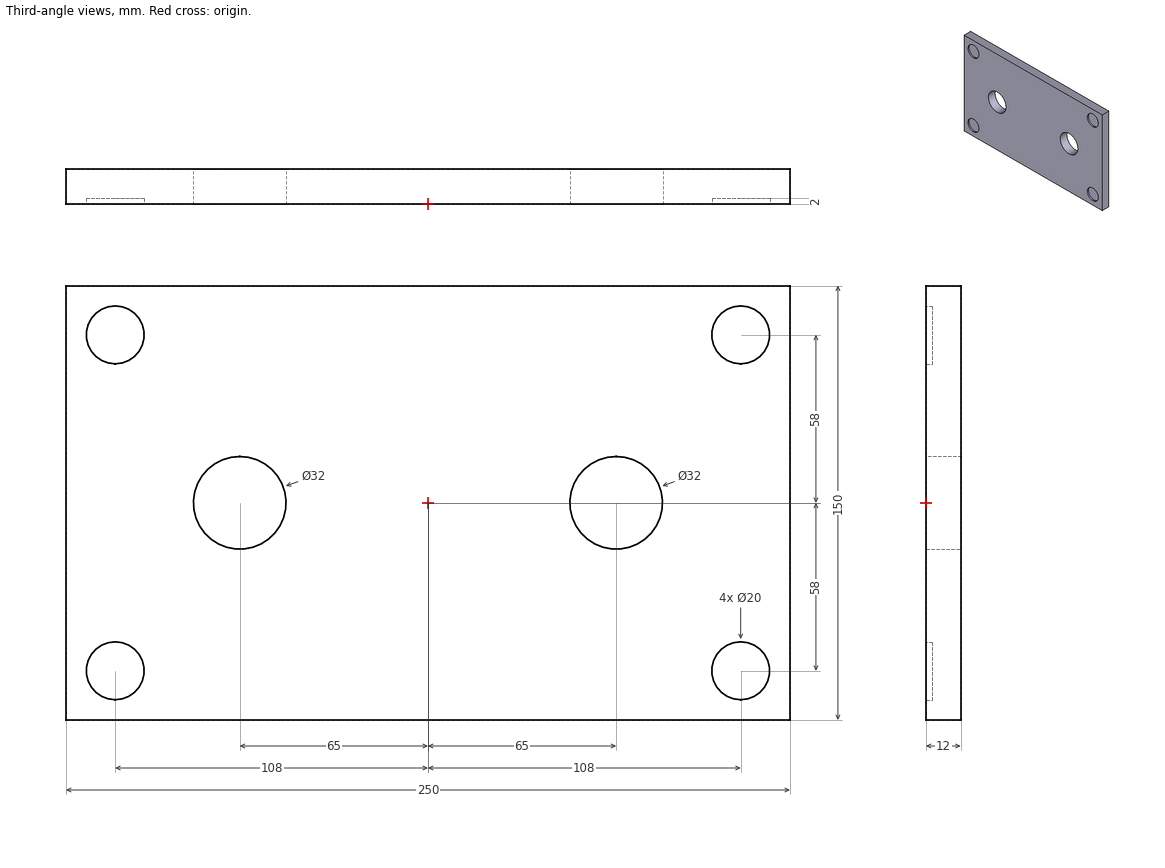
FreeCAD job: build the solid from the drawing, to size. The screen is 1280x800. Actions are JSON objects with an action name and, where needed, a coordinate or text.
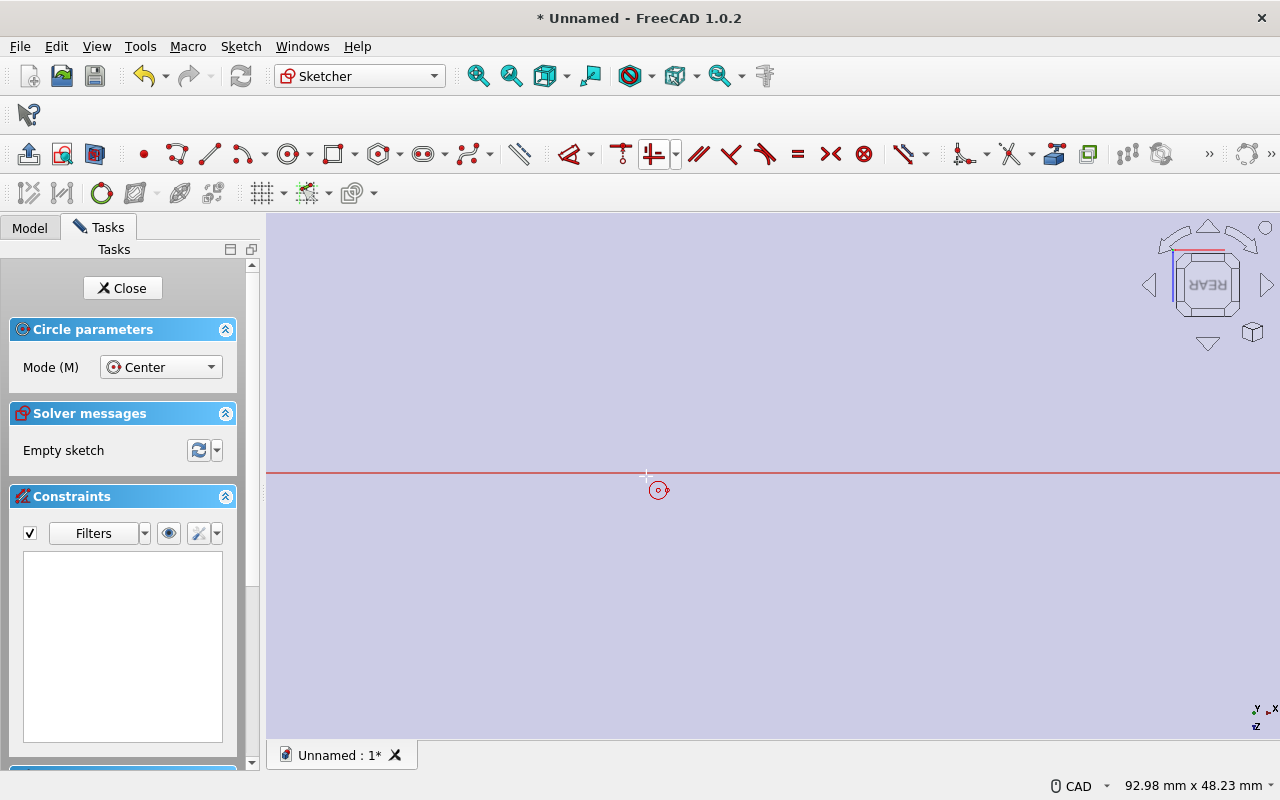
{"action": "left_click", "coordinate": [704, 473]}
{"action": "mouse_move", "coordinate": [827, 350]}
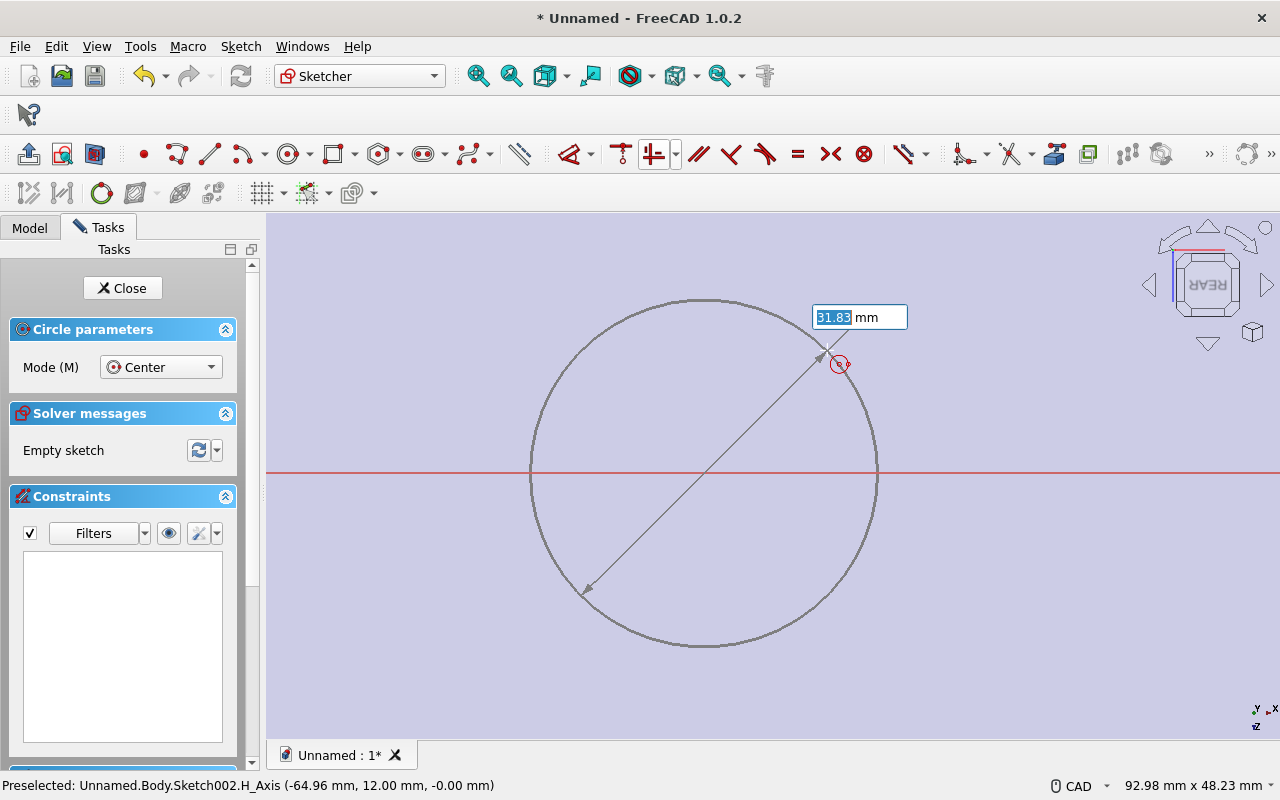
{"action": "type", "text": "32"}
{"action": "key", "text": "Return"}
{"action": "key", "text": "Escape"}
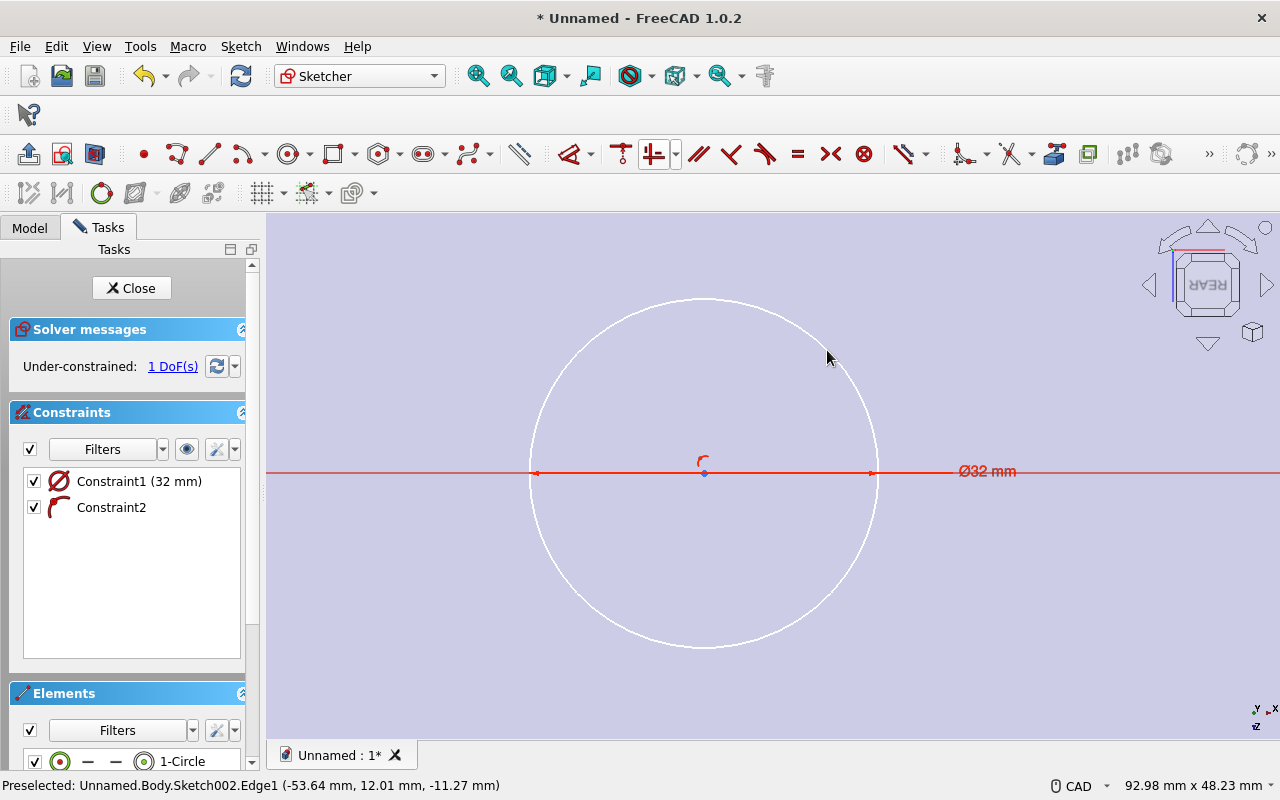
{"action": "left_click", "coordinate": [568, 154]}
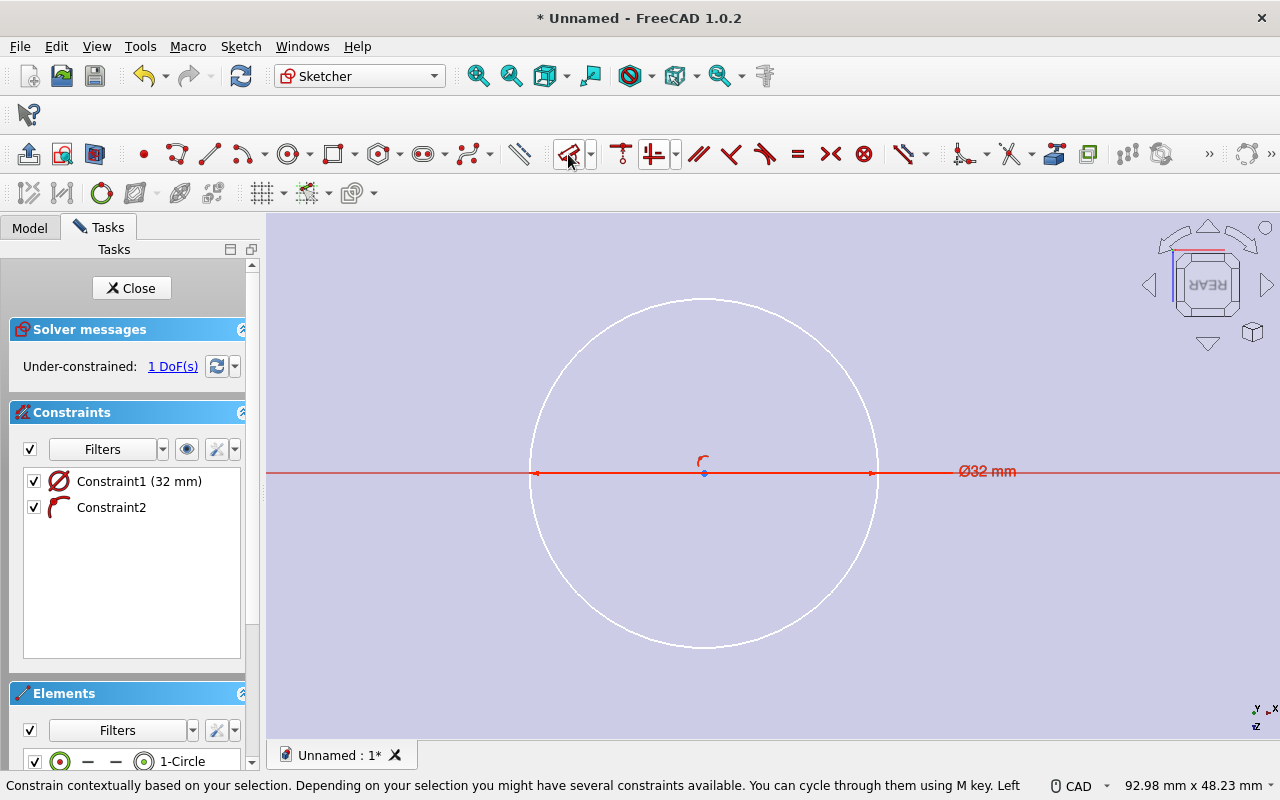
{"action": "left_click", "coordinate": [704, 473]}
{"action": "left_click", "coordinate": [909, 507]}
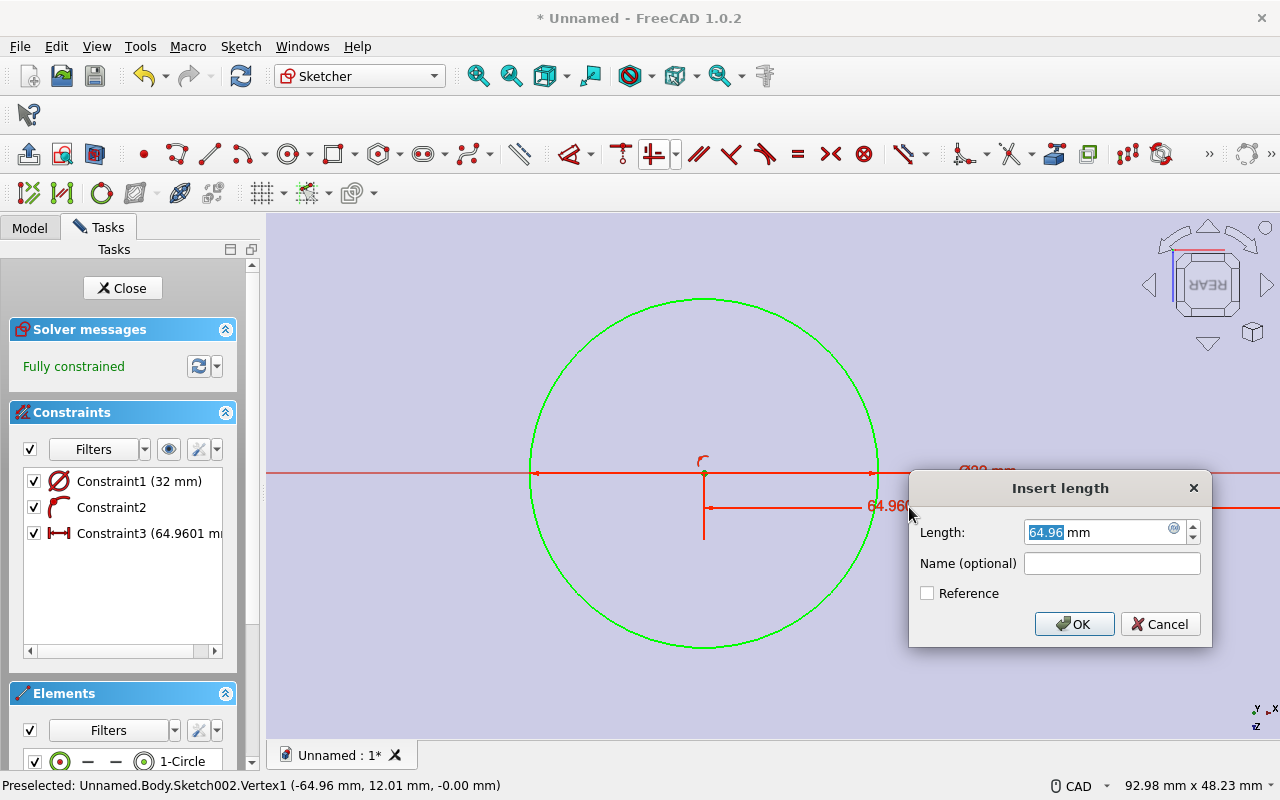
{"action": "type", "text": "65"}
{"action": "key", "text": "Return"}
{"action": "key", "text": "Escape"}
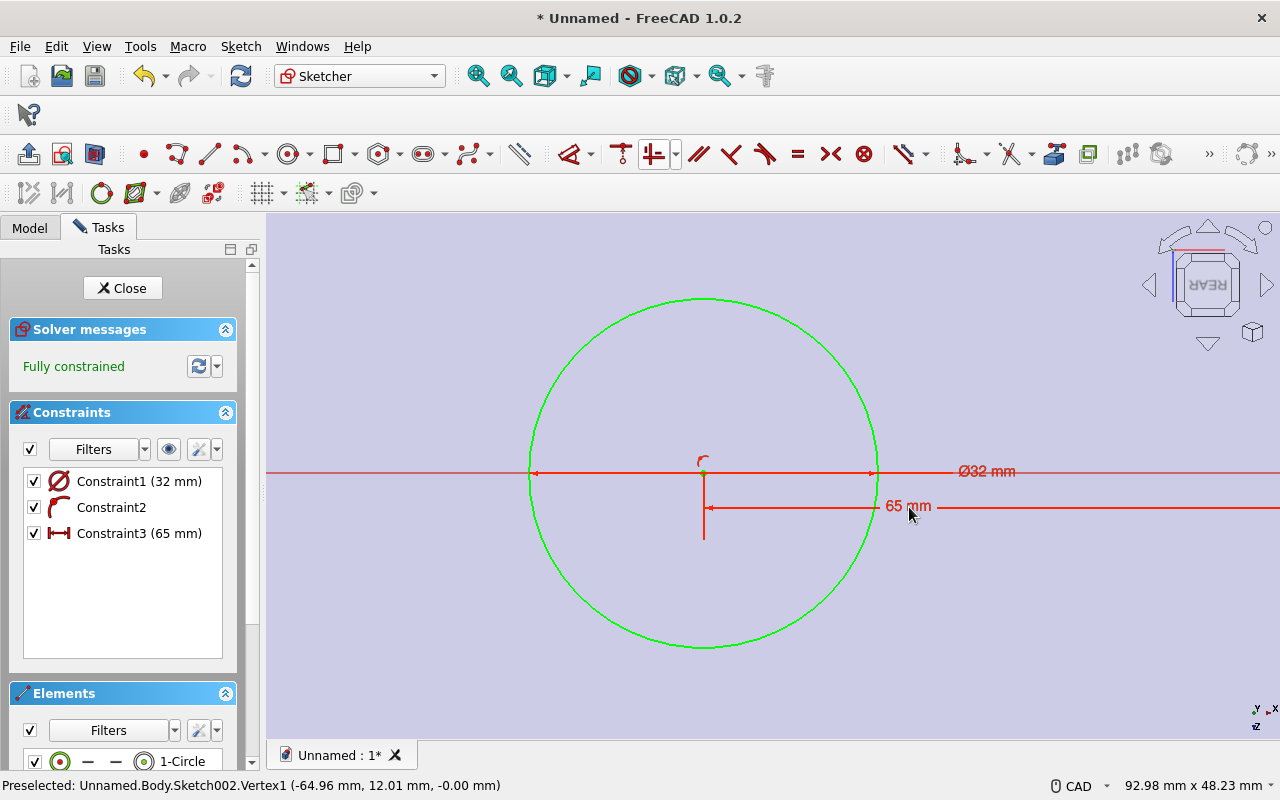
{"action": "left_click", "coordinate": [123, 288]}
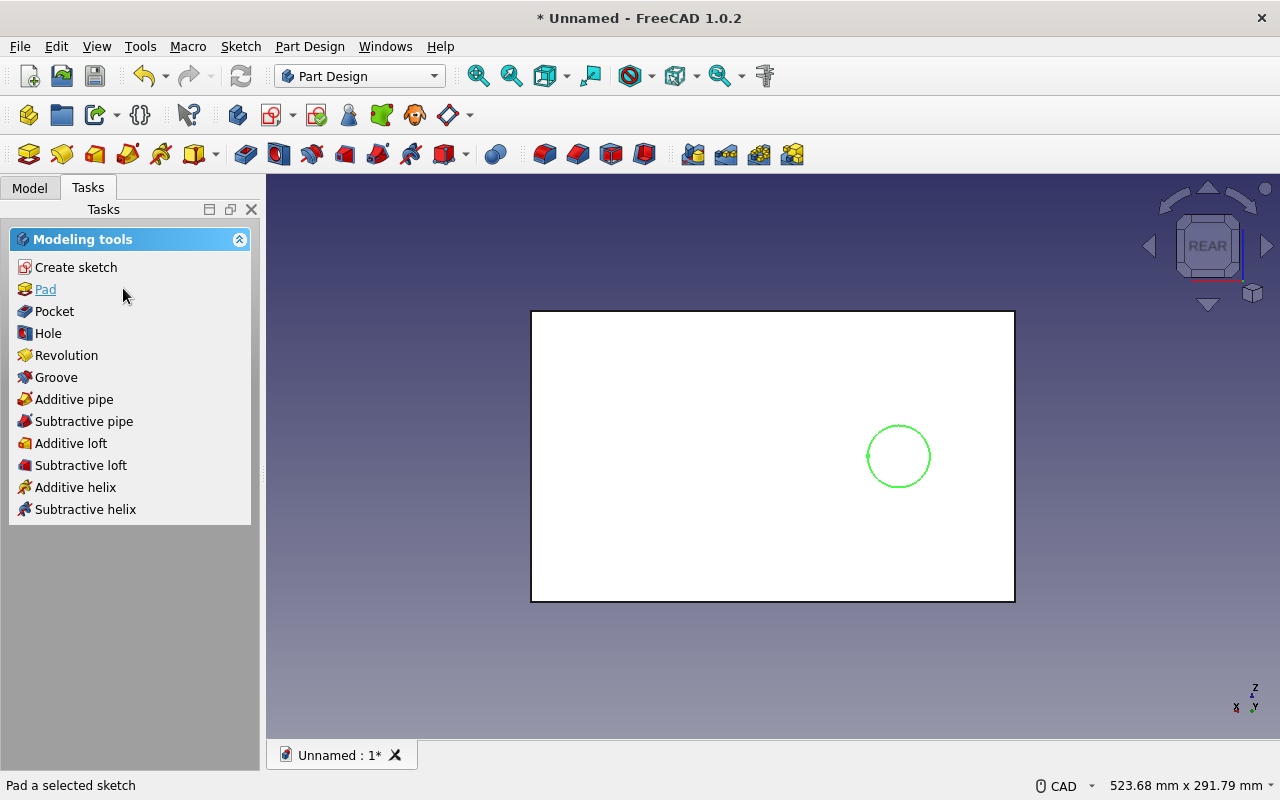
{"action": "left_click", "coordinate": [246, 154]}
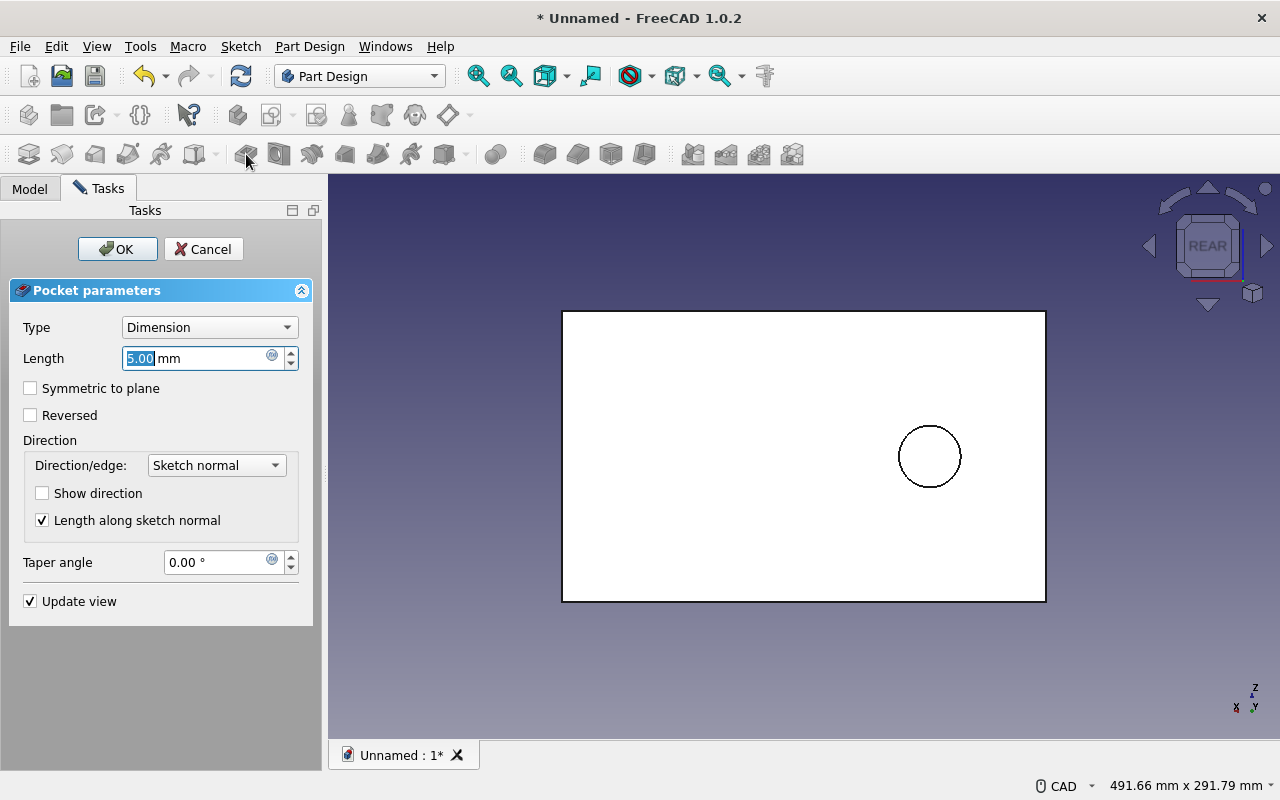
{"action": "left_click", "coordinate": [210, 328]}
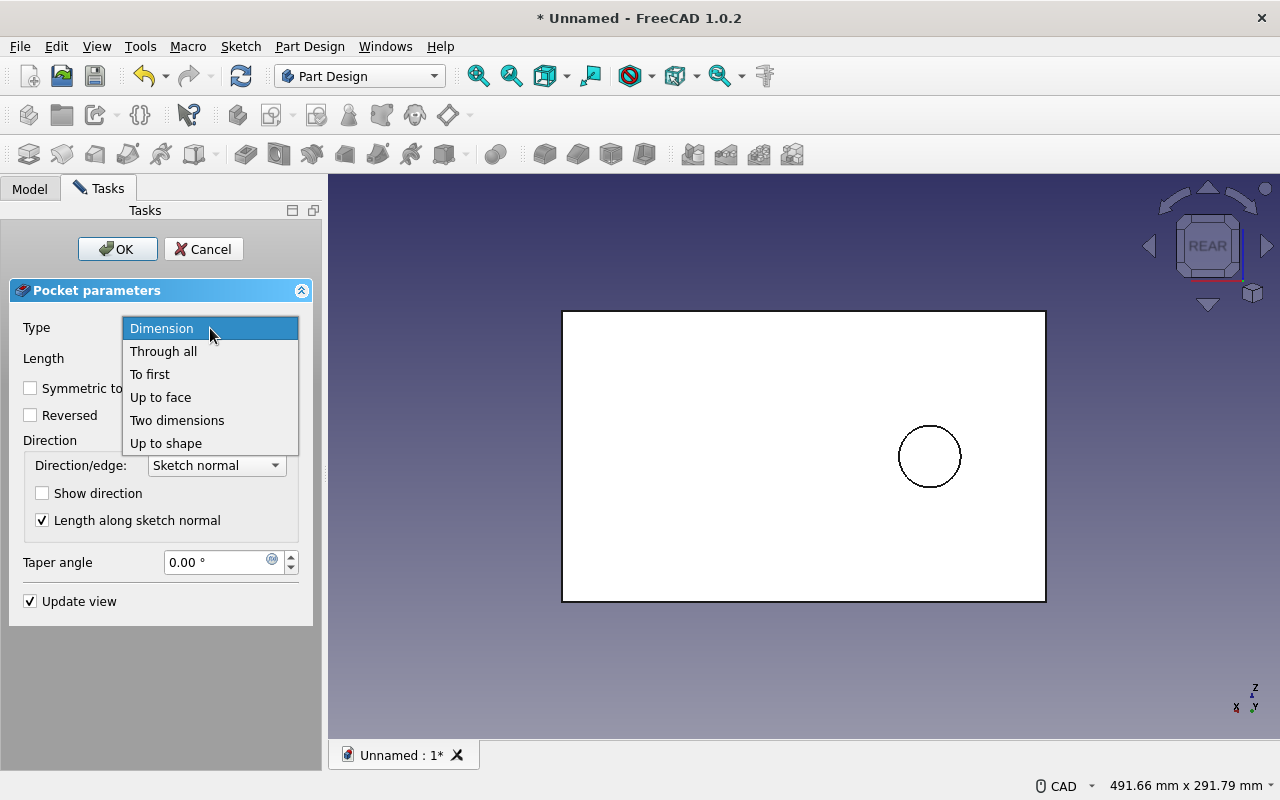
{"action": "left_click", "coordinate": [208, 374]}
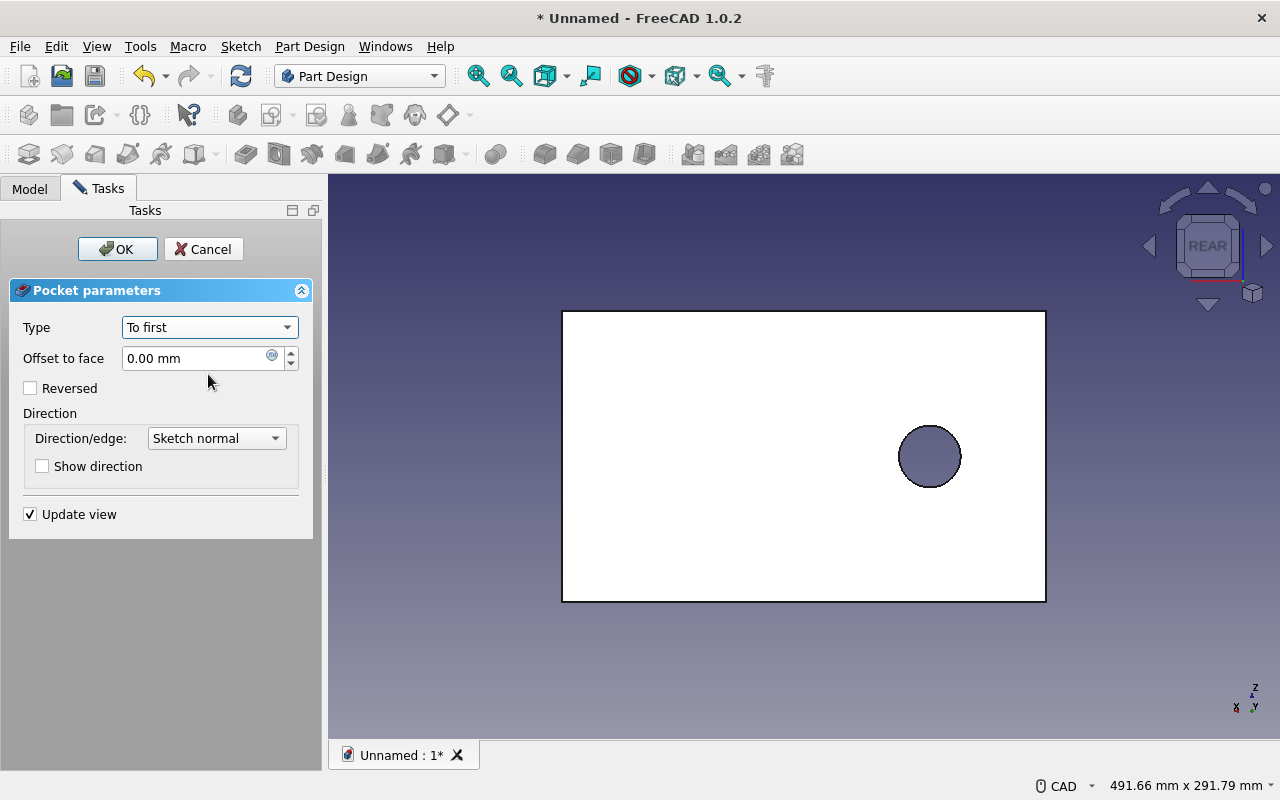
{"action": "left_click", "coordinate": [118, 249]}